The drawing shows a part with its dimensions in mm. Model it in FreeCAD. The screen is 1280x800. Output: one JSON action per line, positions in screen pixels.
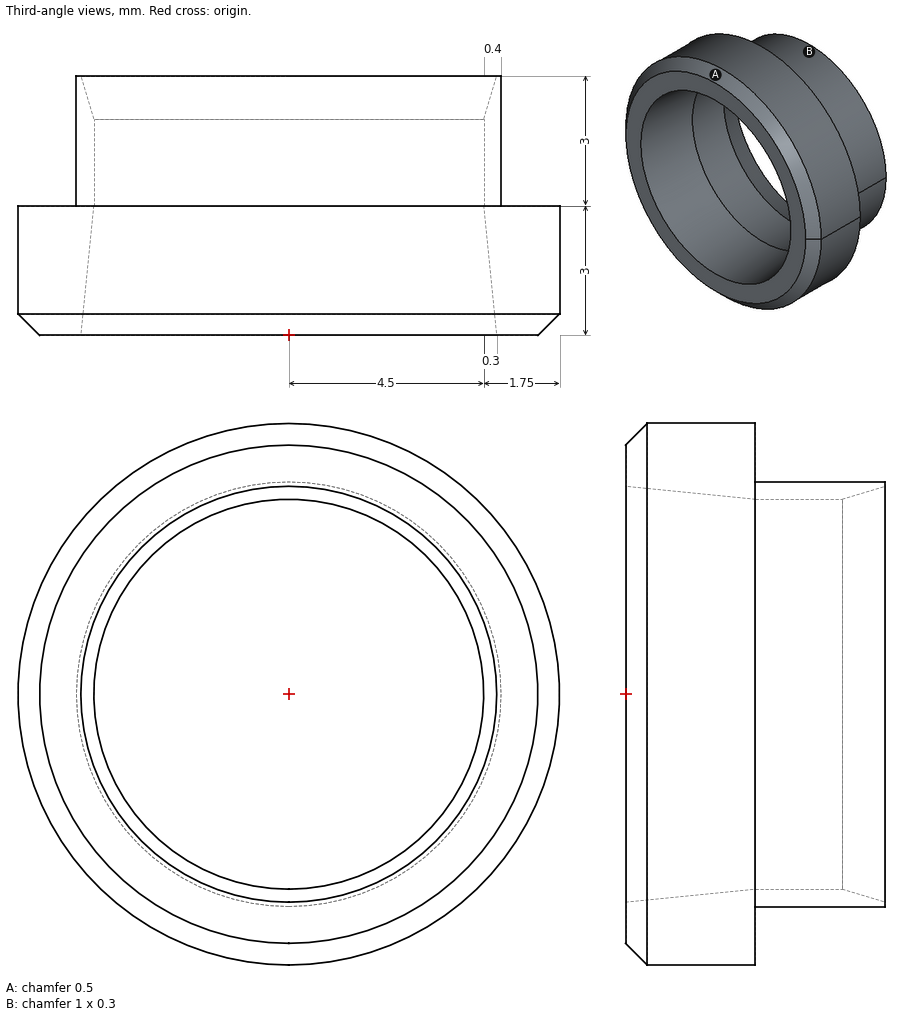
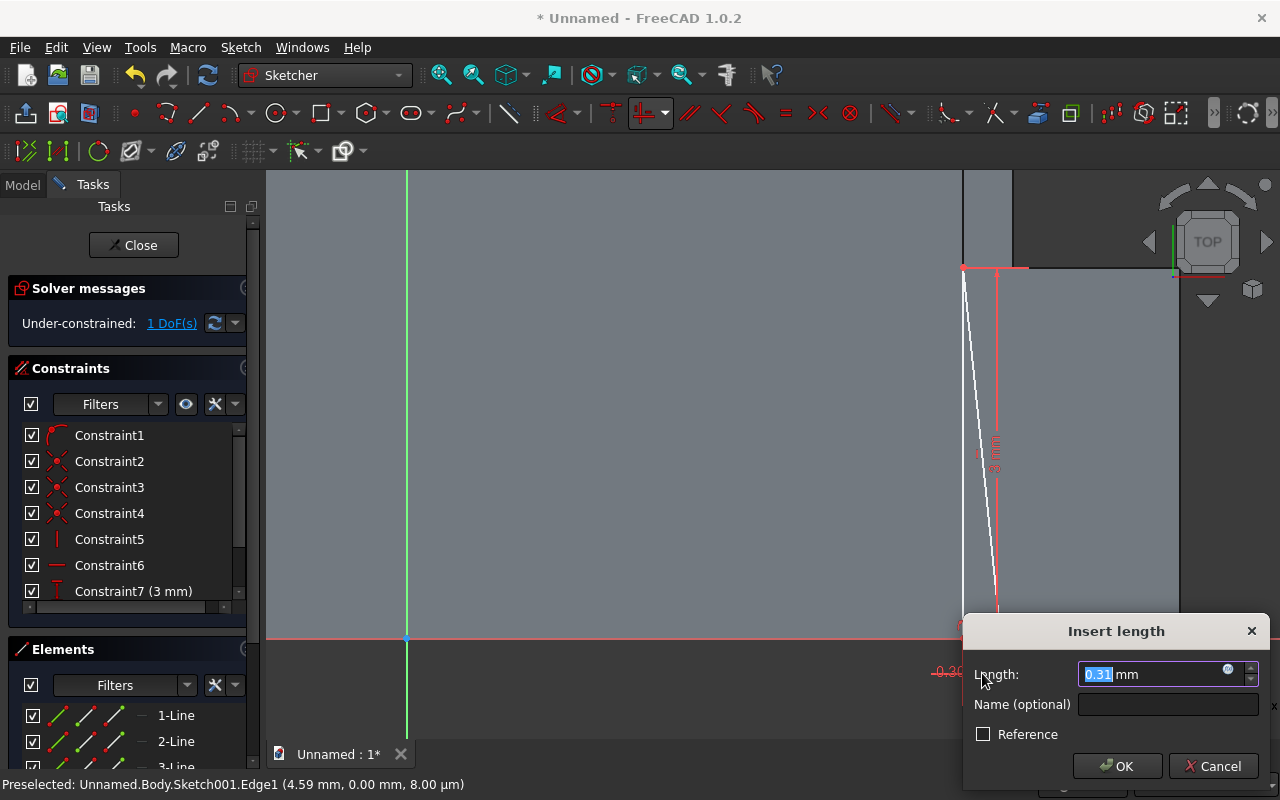
{"action": "type", "text": "0.3"}
{"action": "key", "text": "Return"}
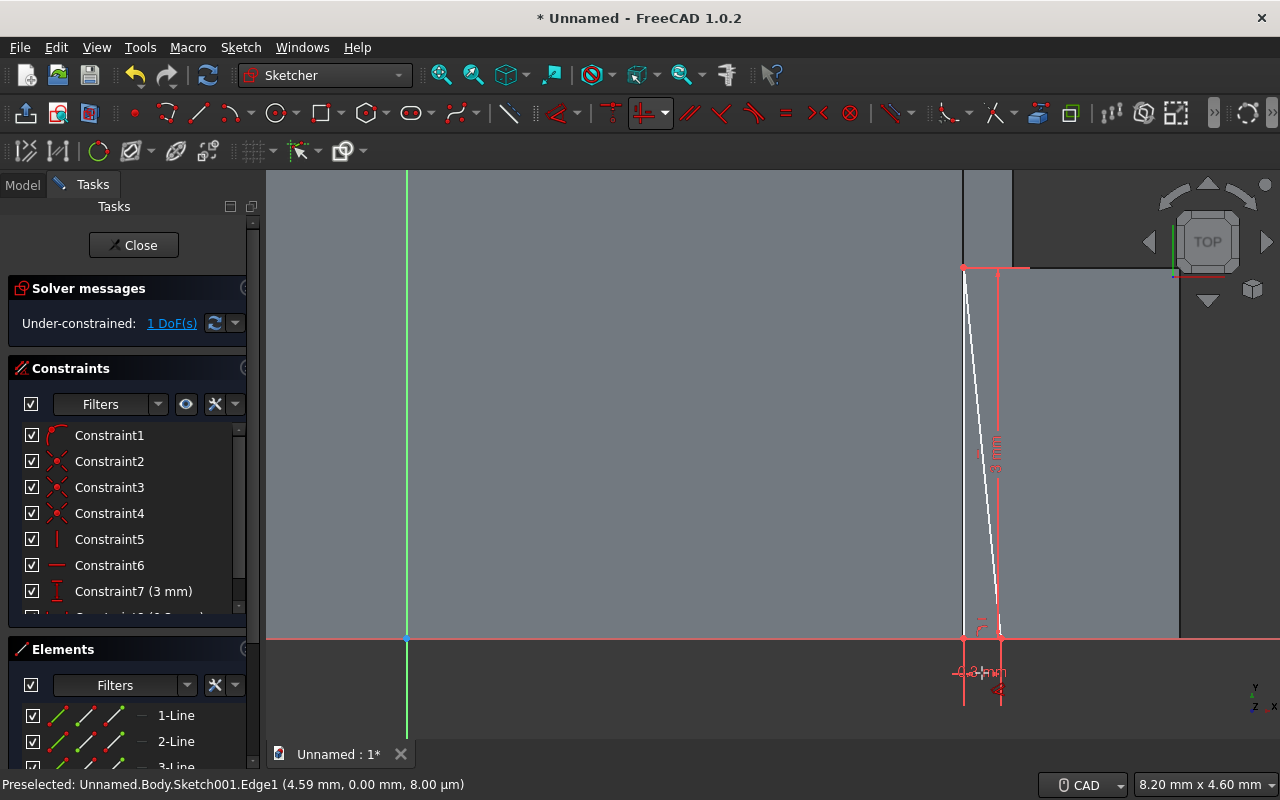
{"action": "left_click", "coordinate": [964, 639]}
{"action": "left_click", "coordinate": [685, 673]}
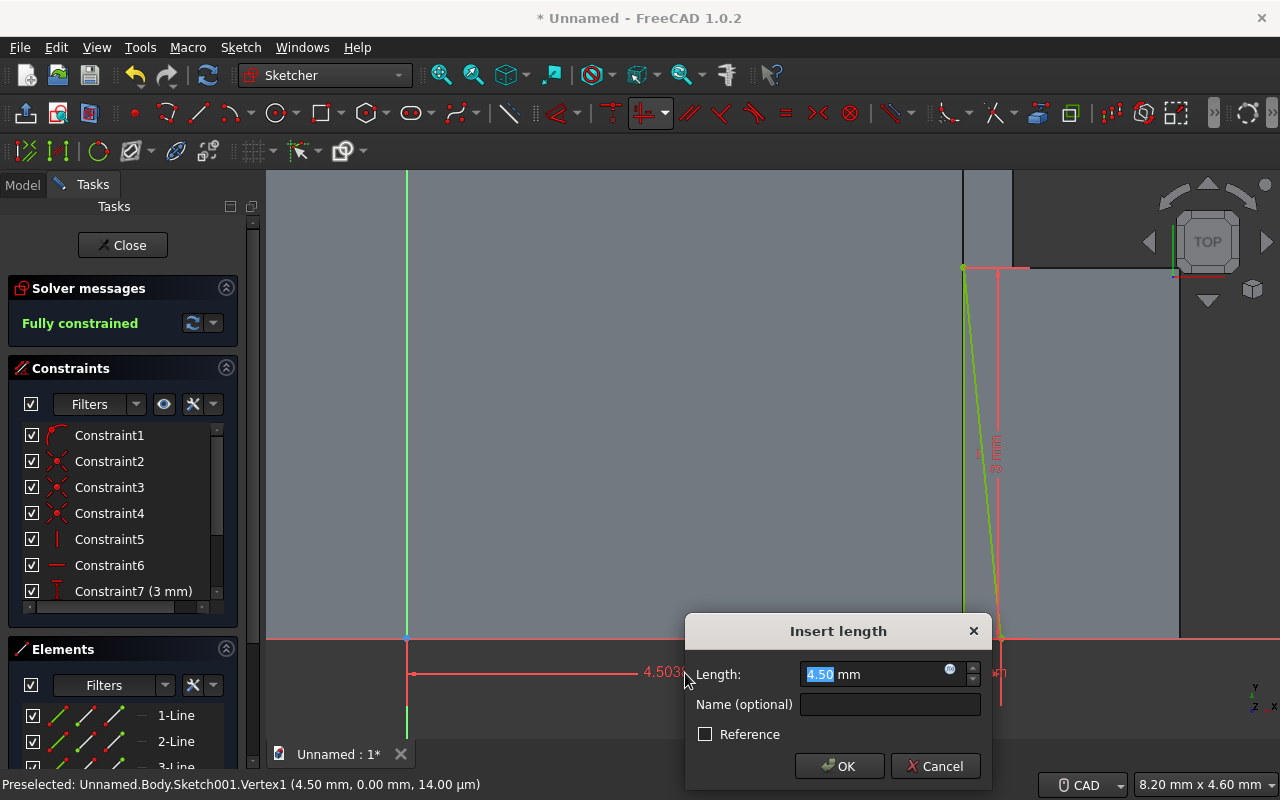
{"action": "type", "text": "4.5"}
{"action": "key", "text": "Return"}
{"action": "key", "text": "Escape"}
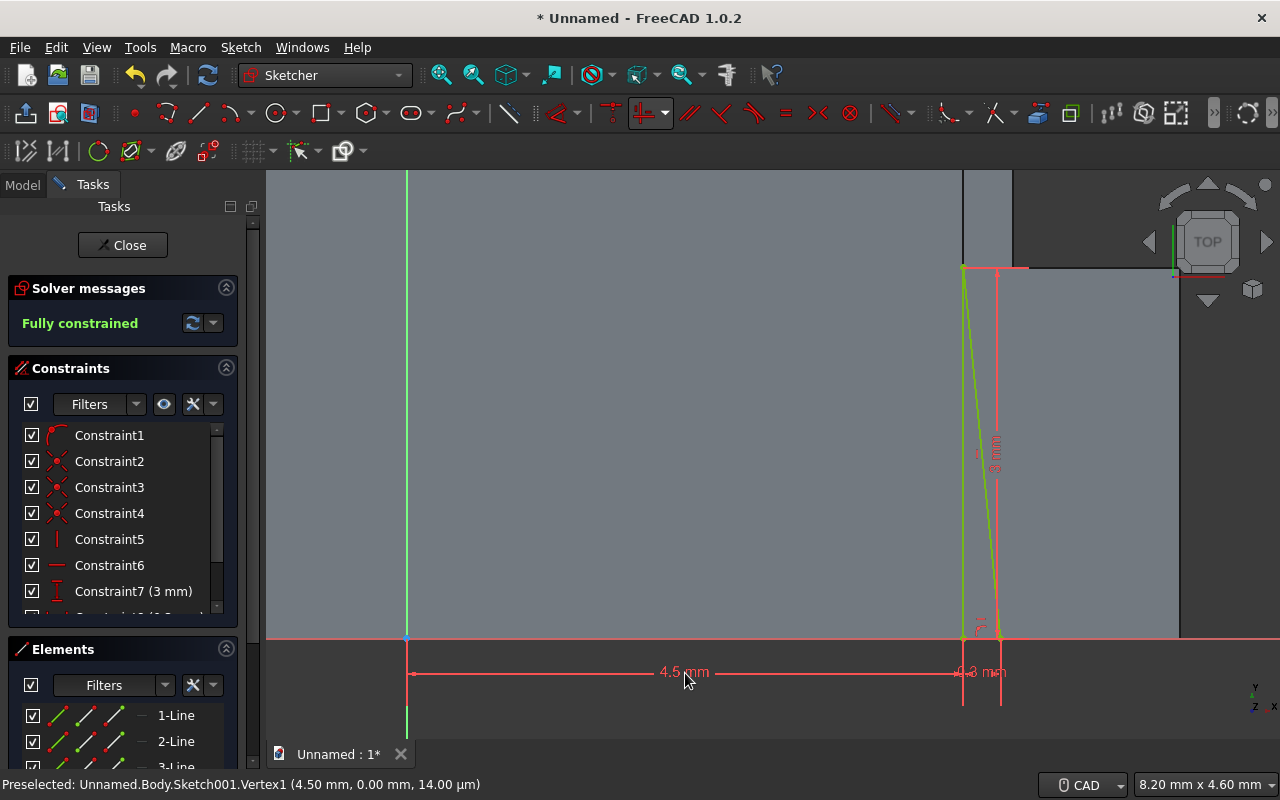
{"action": "left_click", "coordinate": [123, 245]}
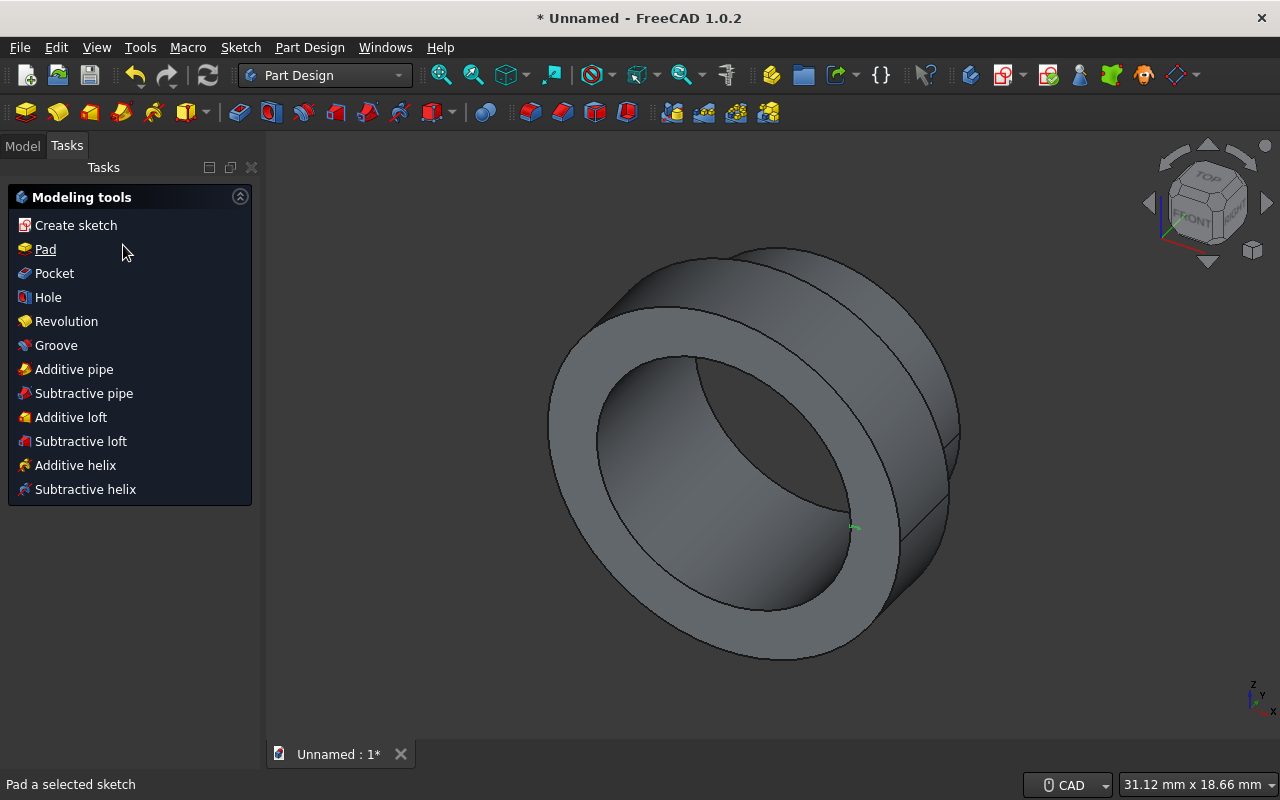
{"action": "left_click", "coordinate": [304, 112]}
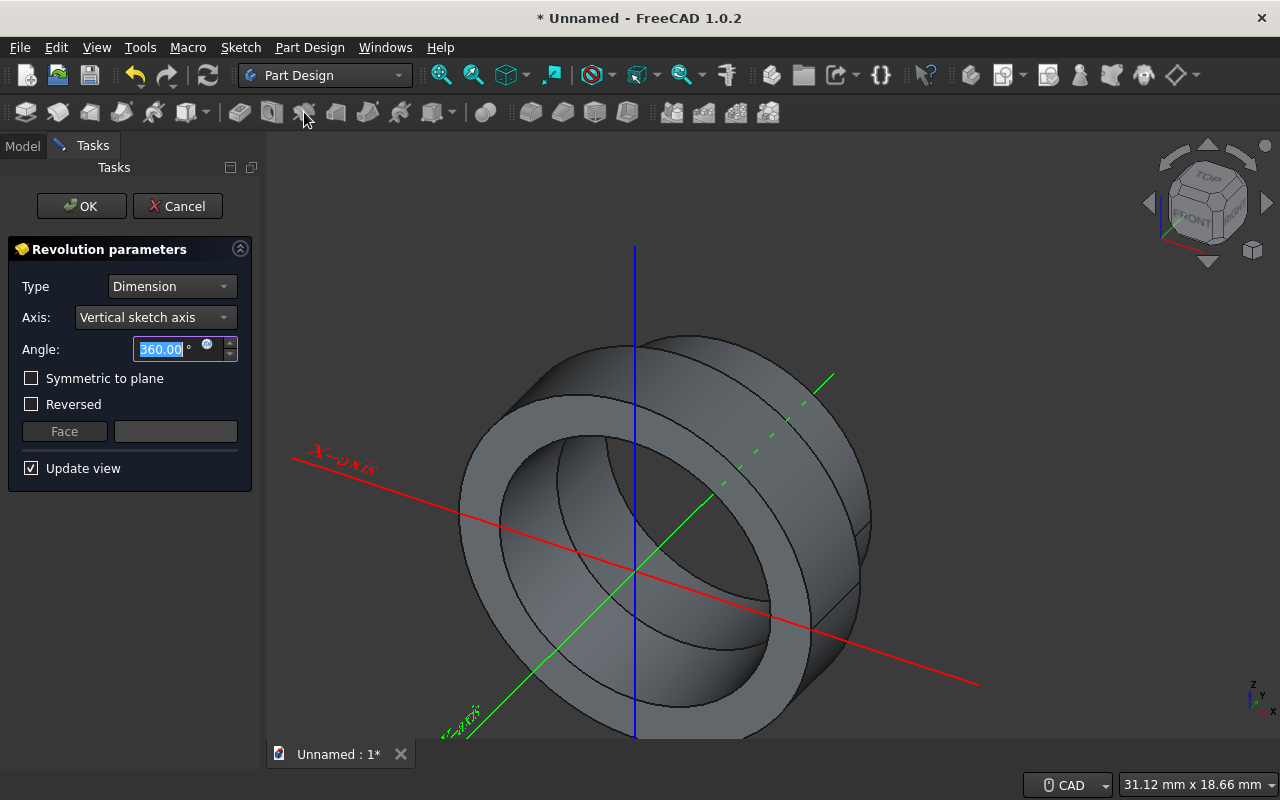
{"action": "left_click", "coordinate": [82, 206]}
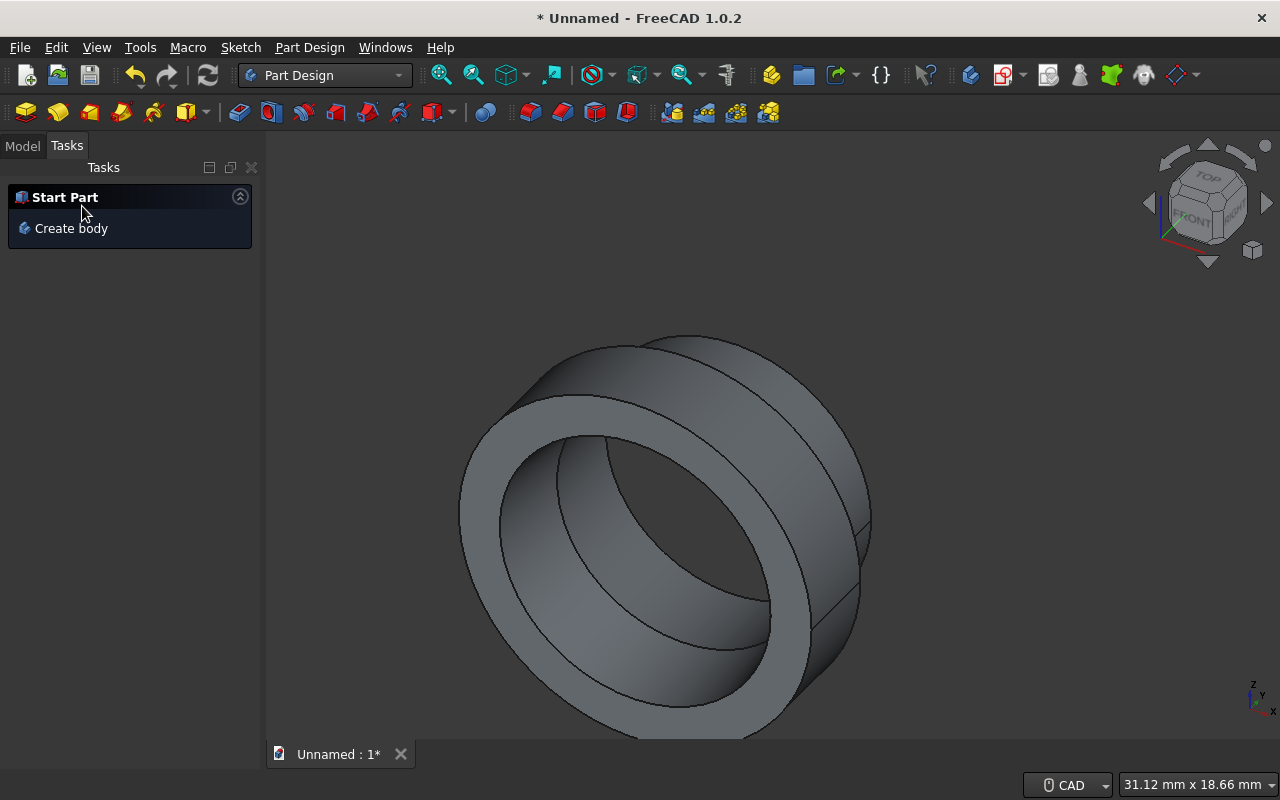
{"action": "left_click", "coordinate": [442, 76]}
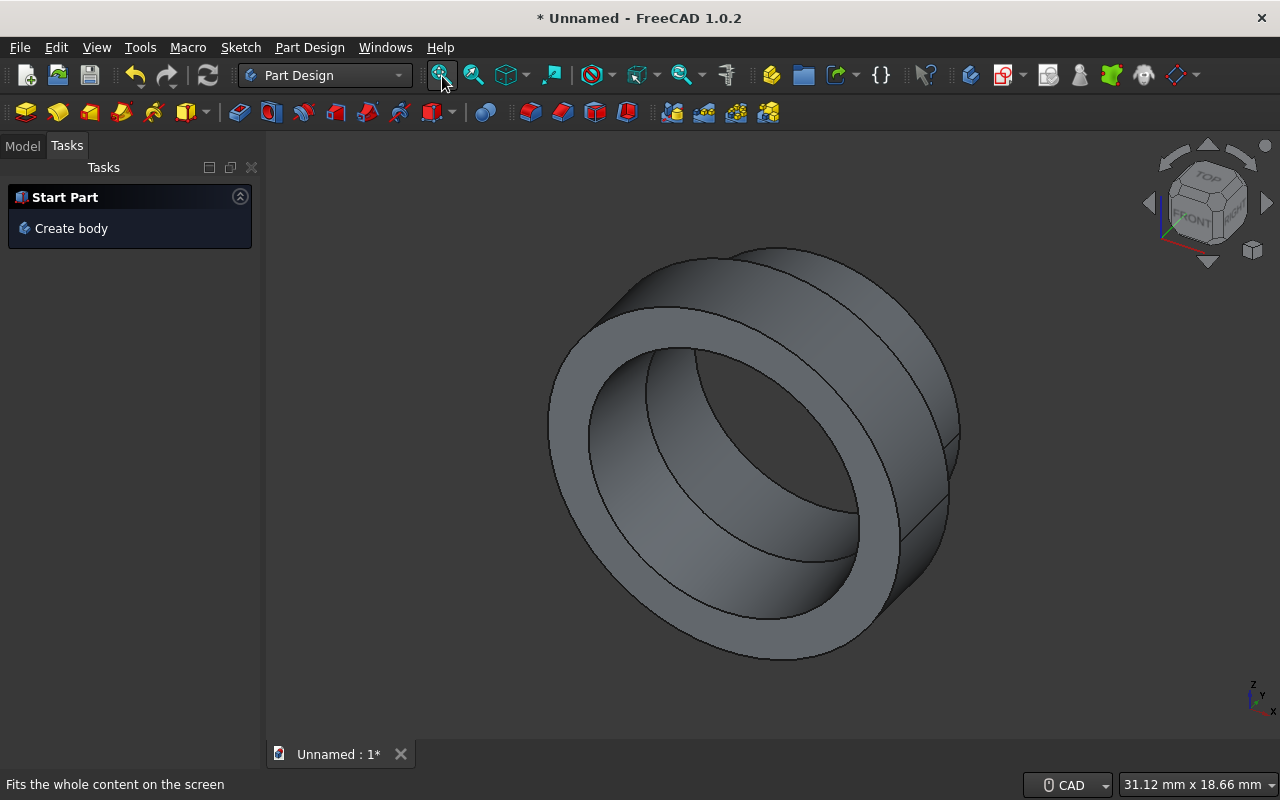
{"action": "left_click", "coordinate": [581, 337]}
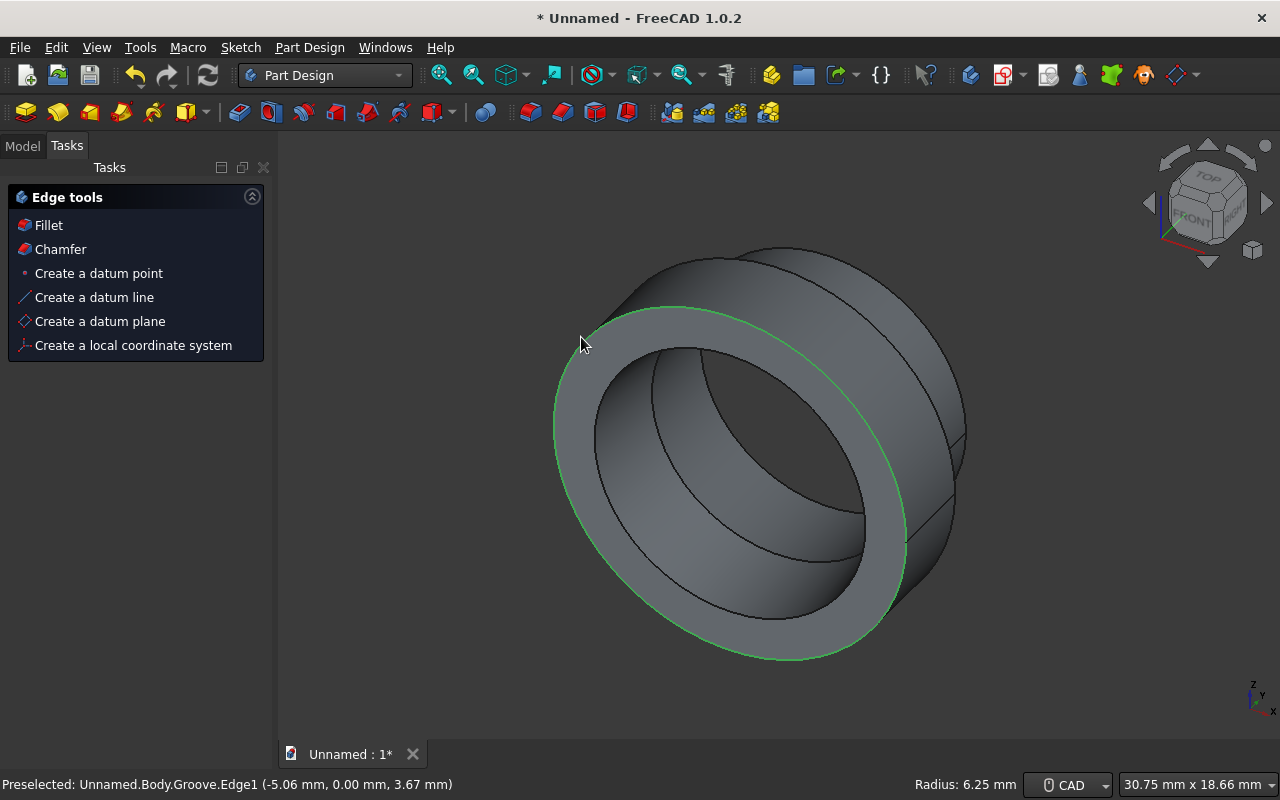
{"action": "left_click", "coordinate": [564, 112]}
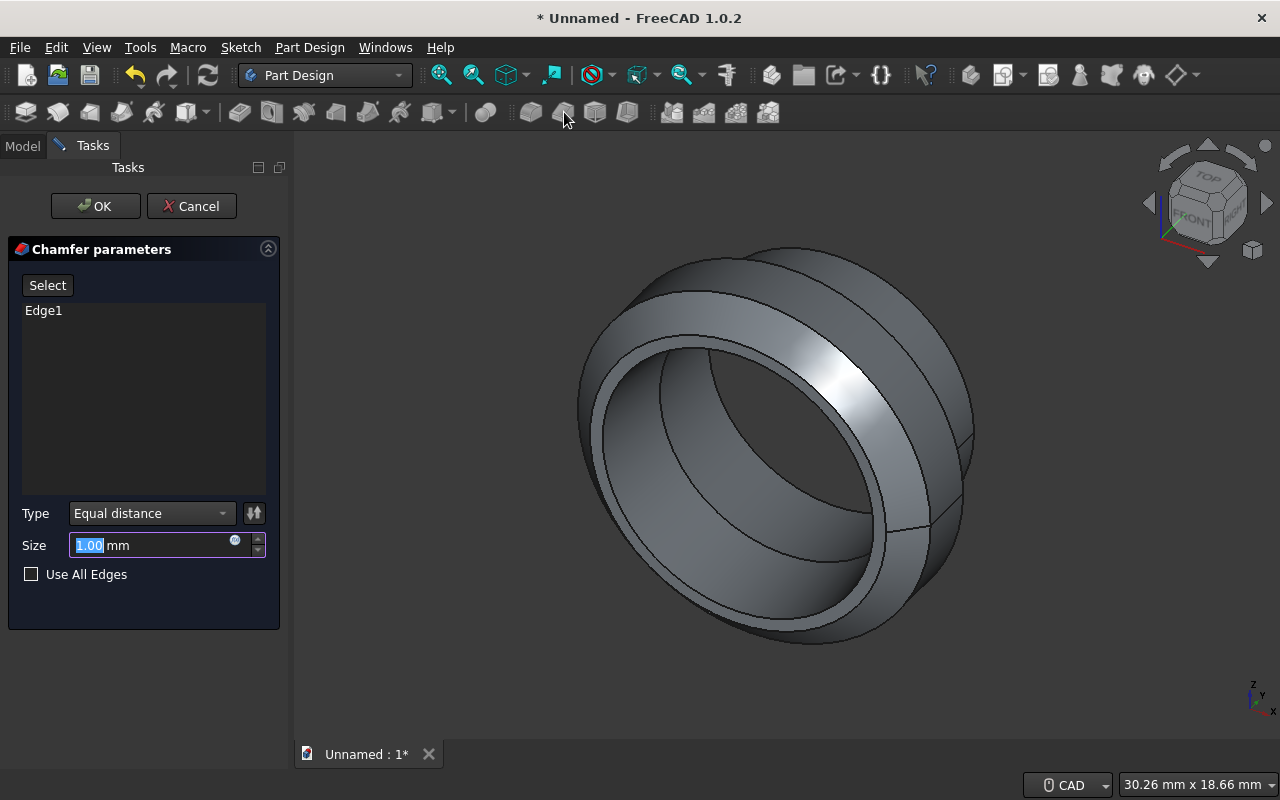
{"action": "type", "text": "0.5"}
{"action": "key", "text": "Tab"}